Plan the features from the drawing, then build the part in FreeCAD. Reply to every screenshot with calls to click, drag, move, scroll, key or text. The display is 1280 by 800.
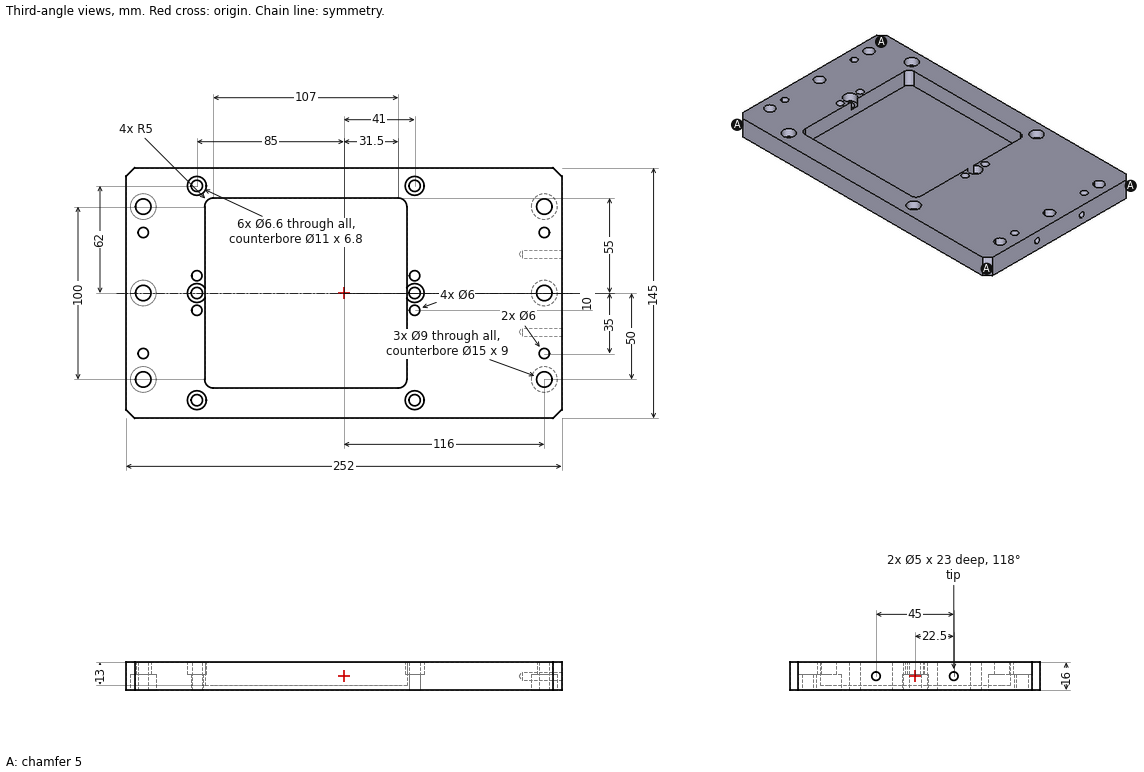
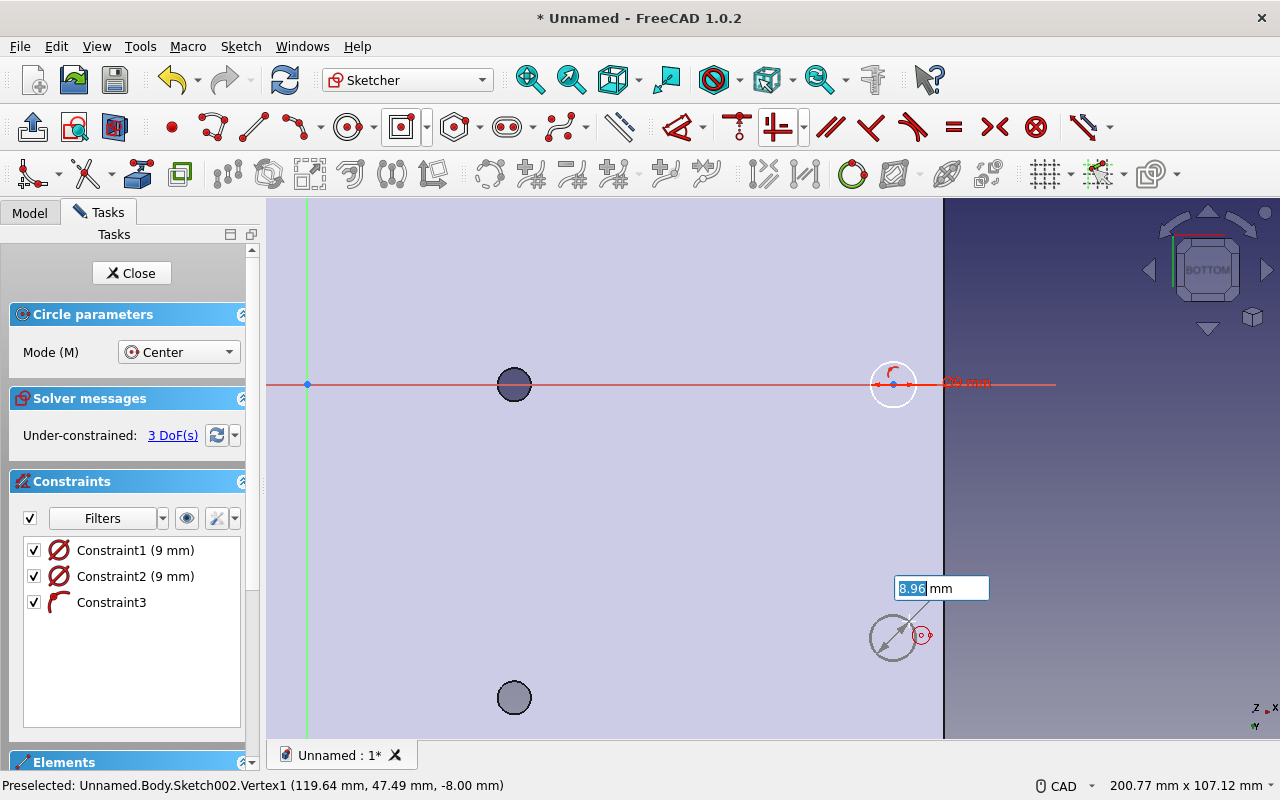
text(9)
key(Return)
key(Escape)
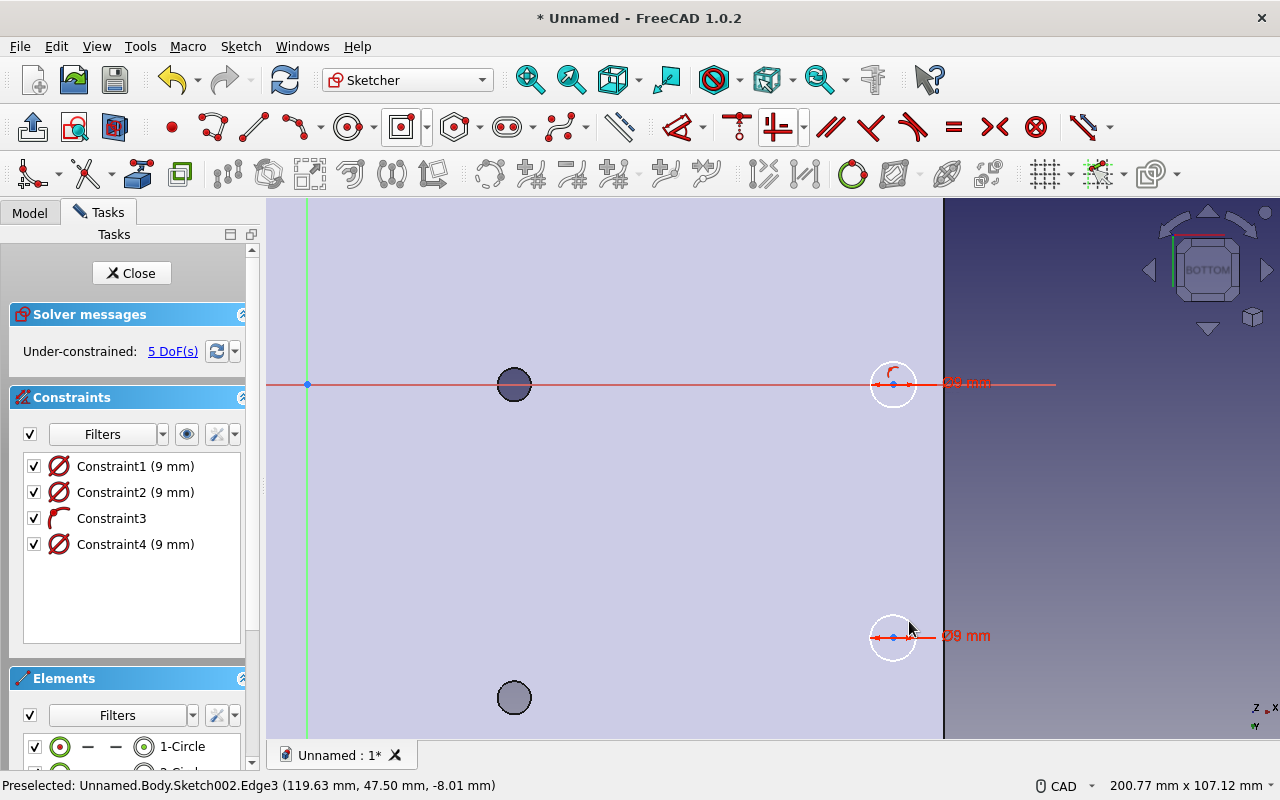
scroll(894, 639, down, 2)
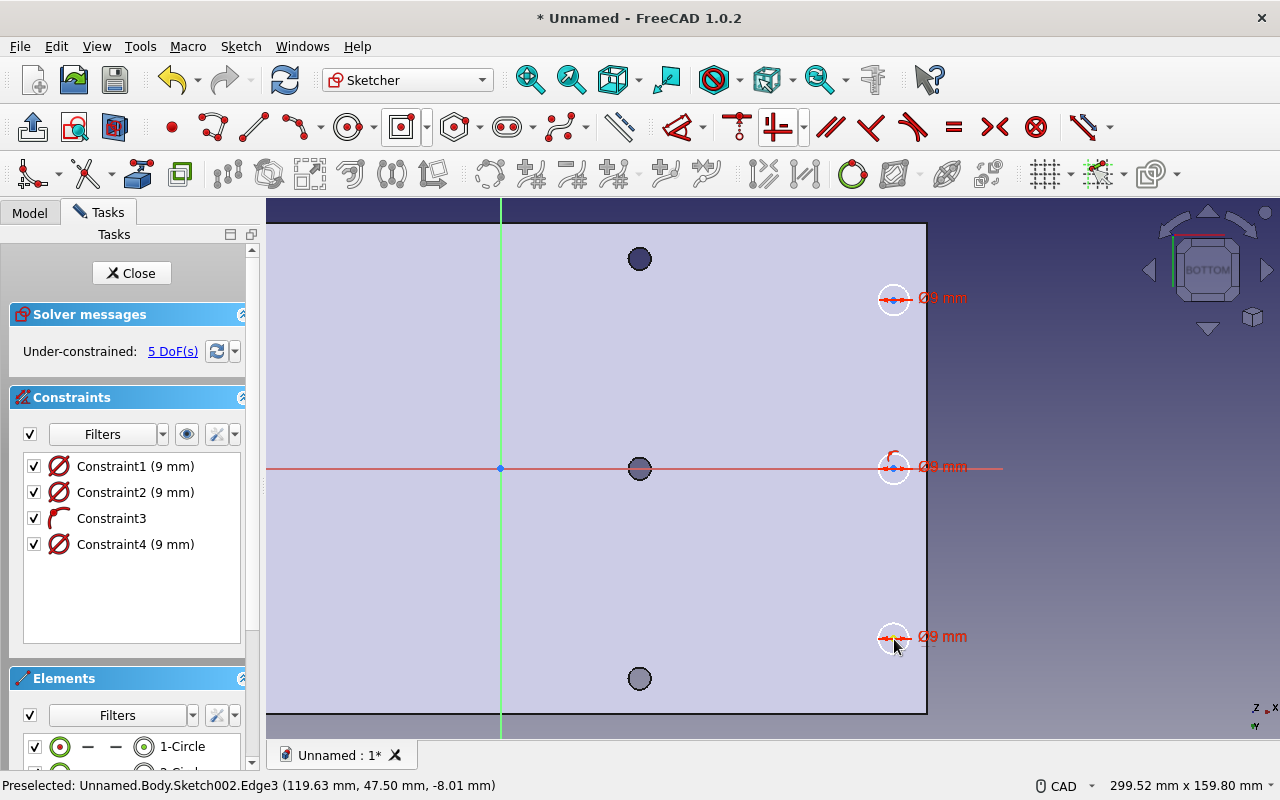
click(894, 300)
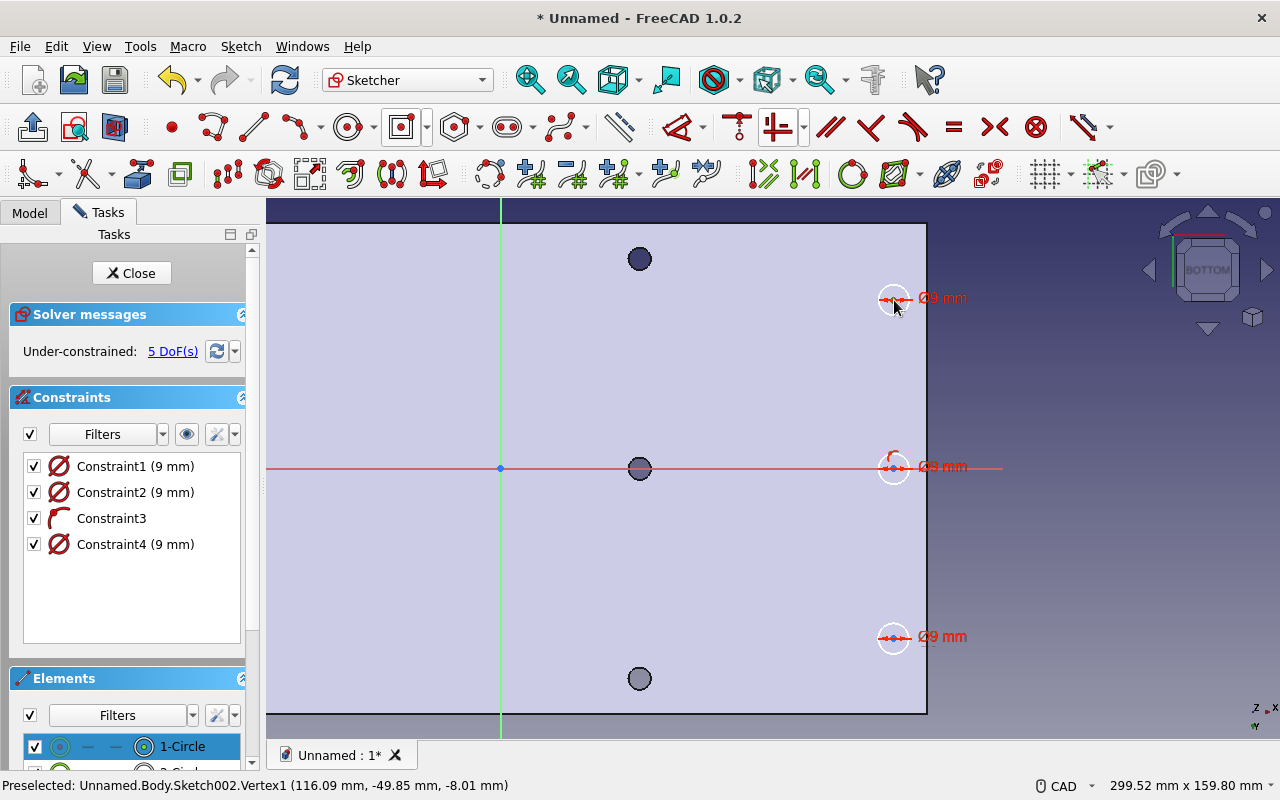
click(894, 639)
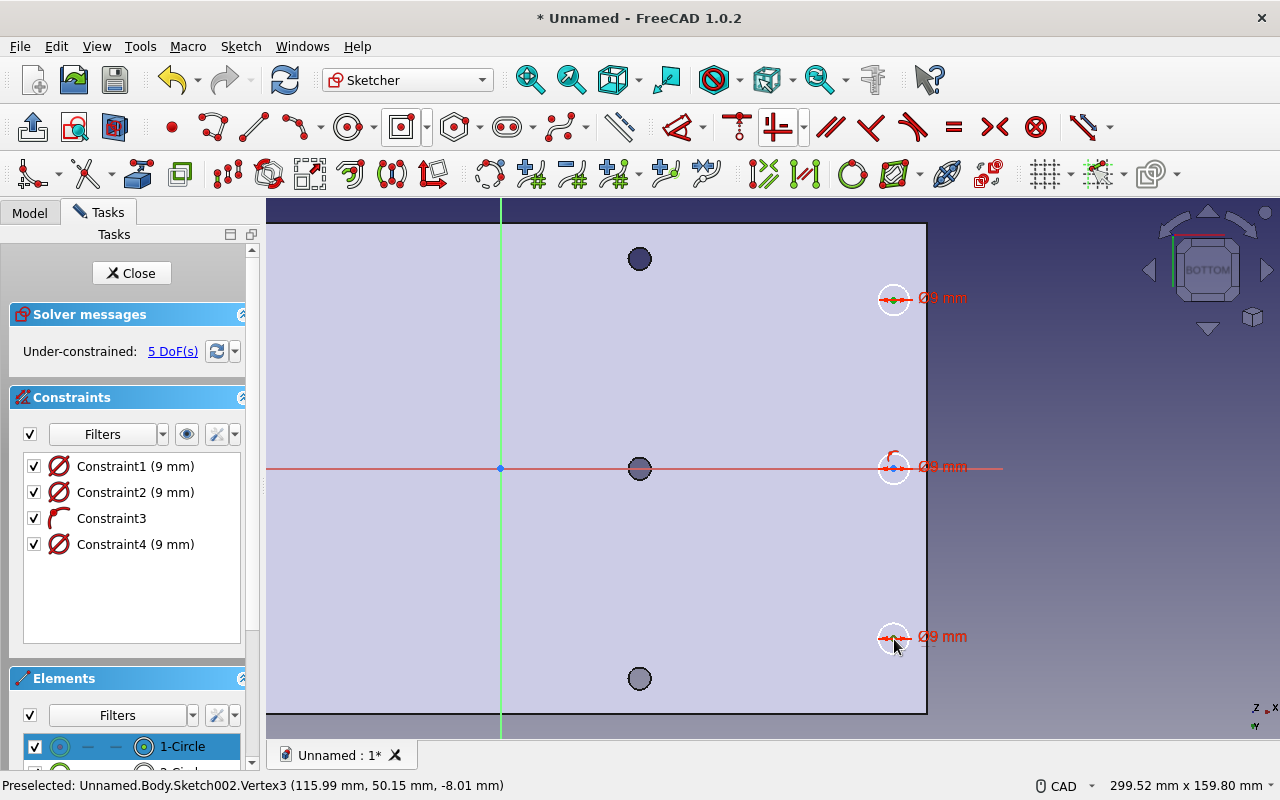
click(353, 469)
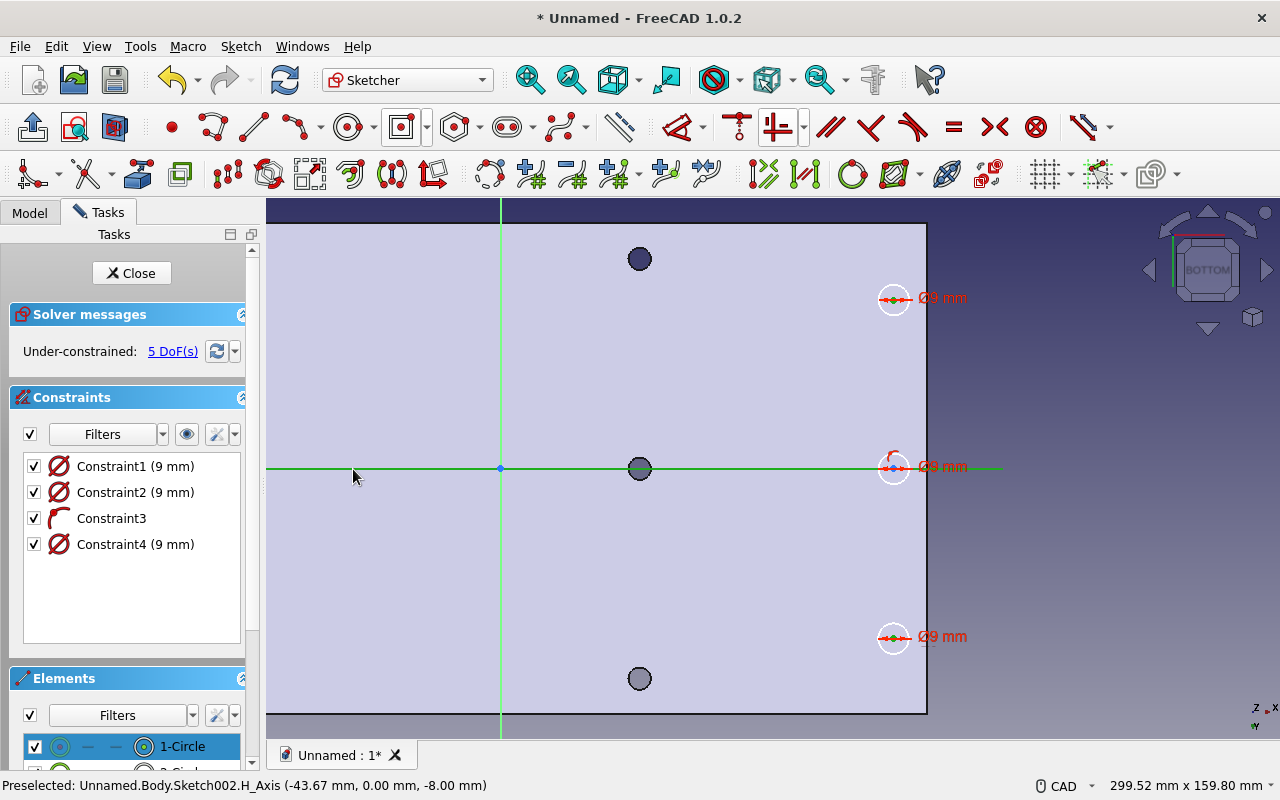
key(s)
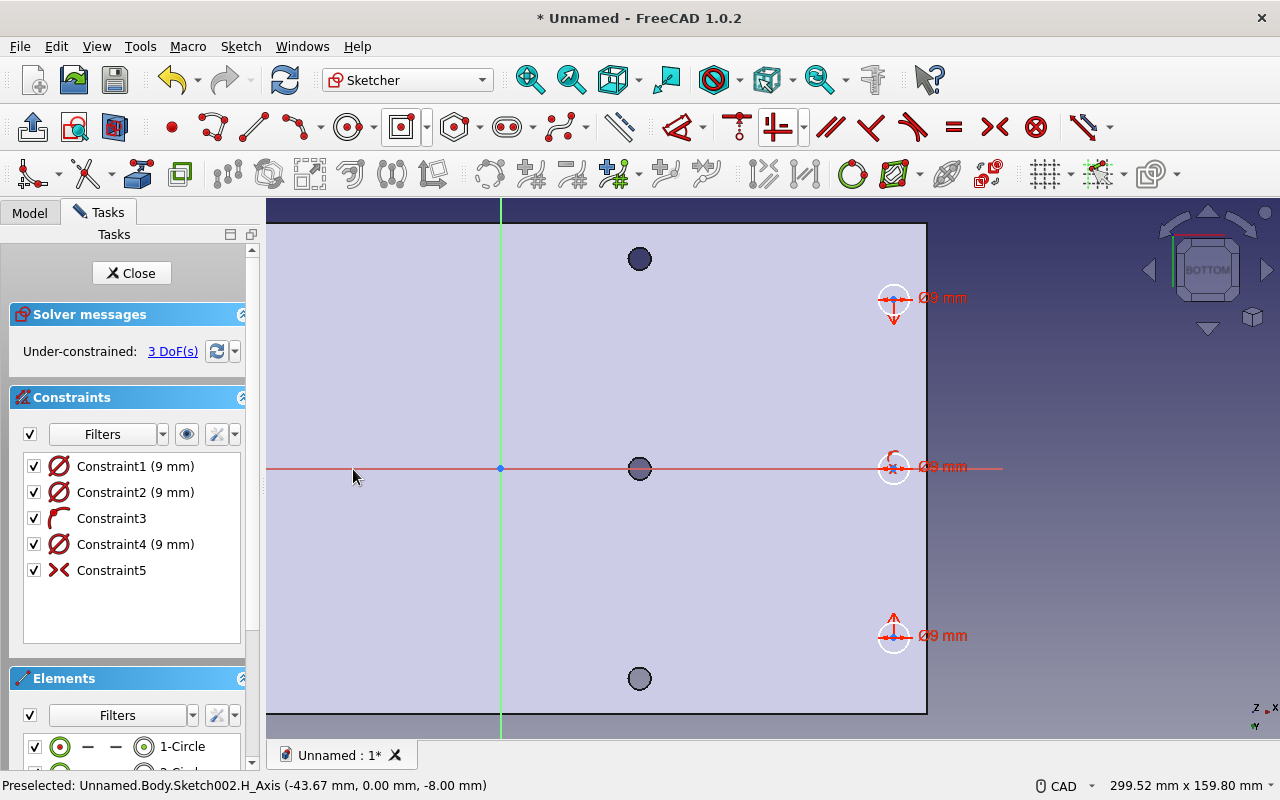
key(d)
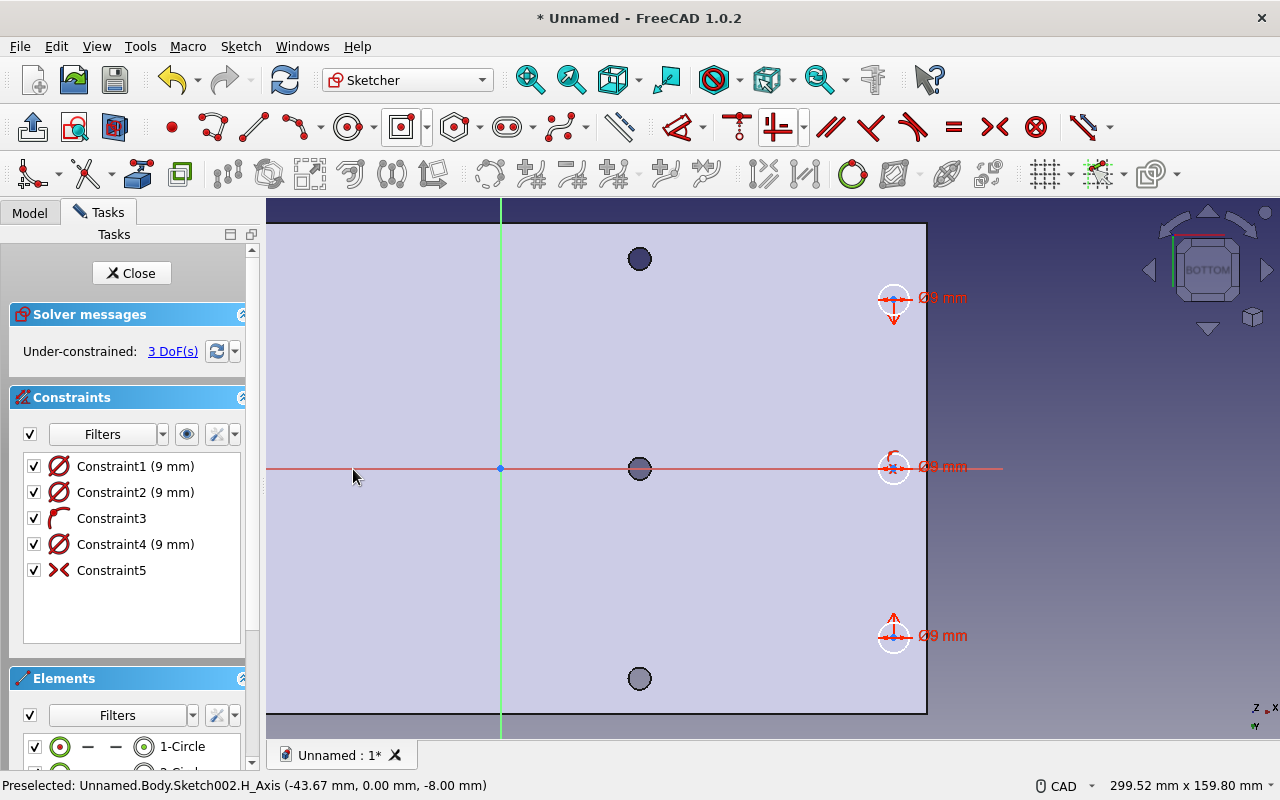
click(894, 300)
click(467, 384)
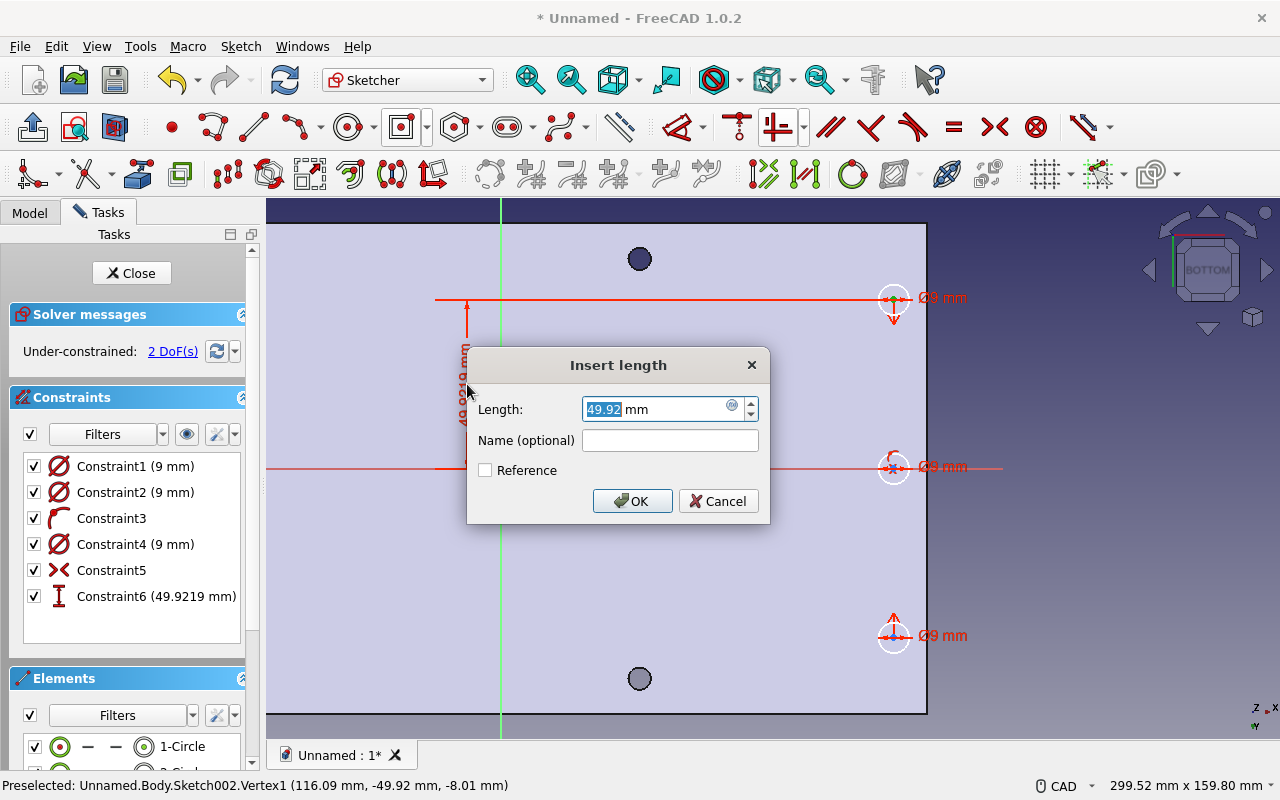
text(50)
key(Return)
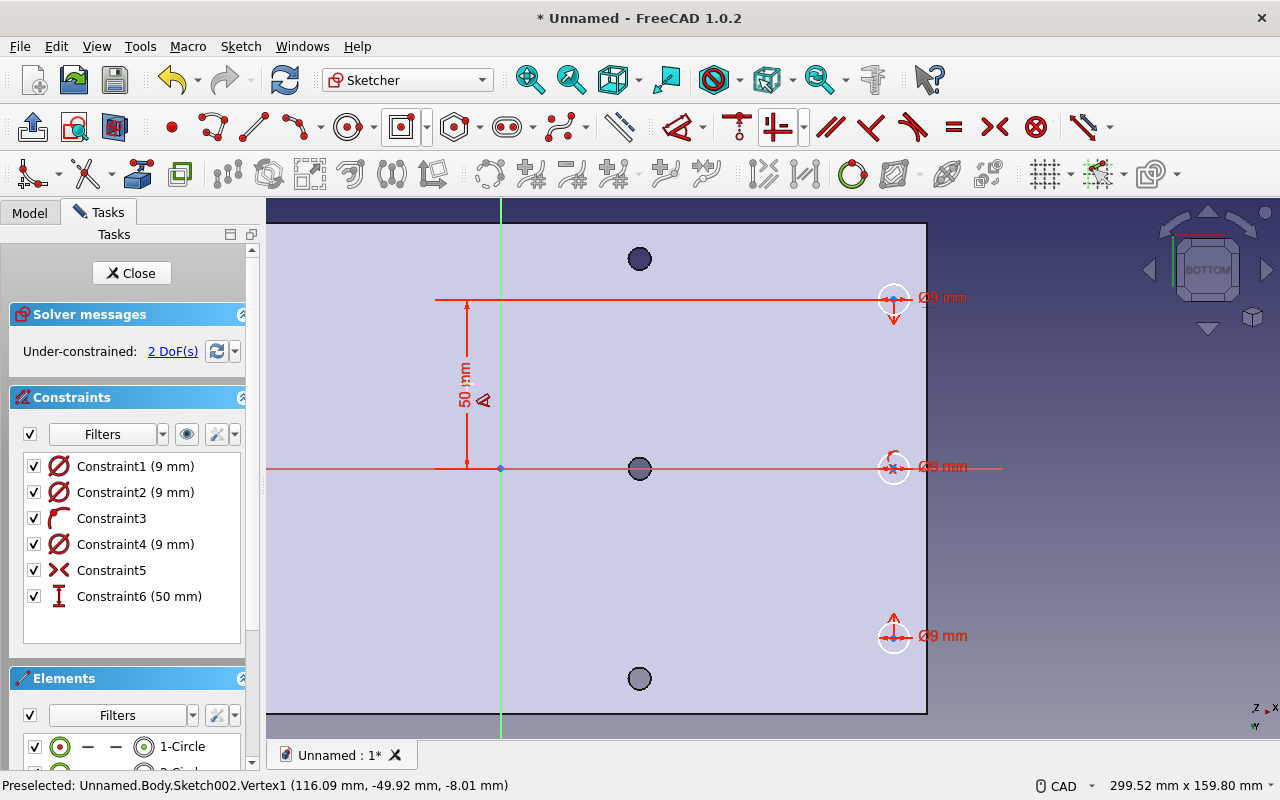
click(894, 300)
click(697, 266)